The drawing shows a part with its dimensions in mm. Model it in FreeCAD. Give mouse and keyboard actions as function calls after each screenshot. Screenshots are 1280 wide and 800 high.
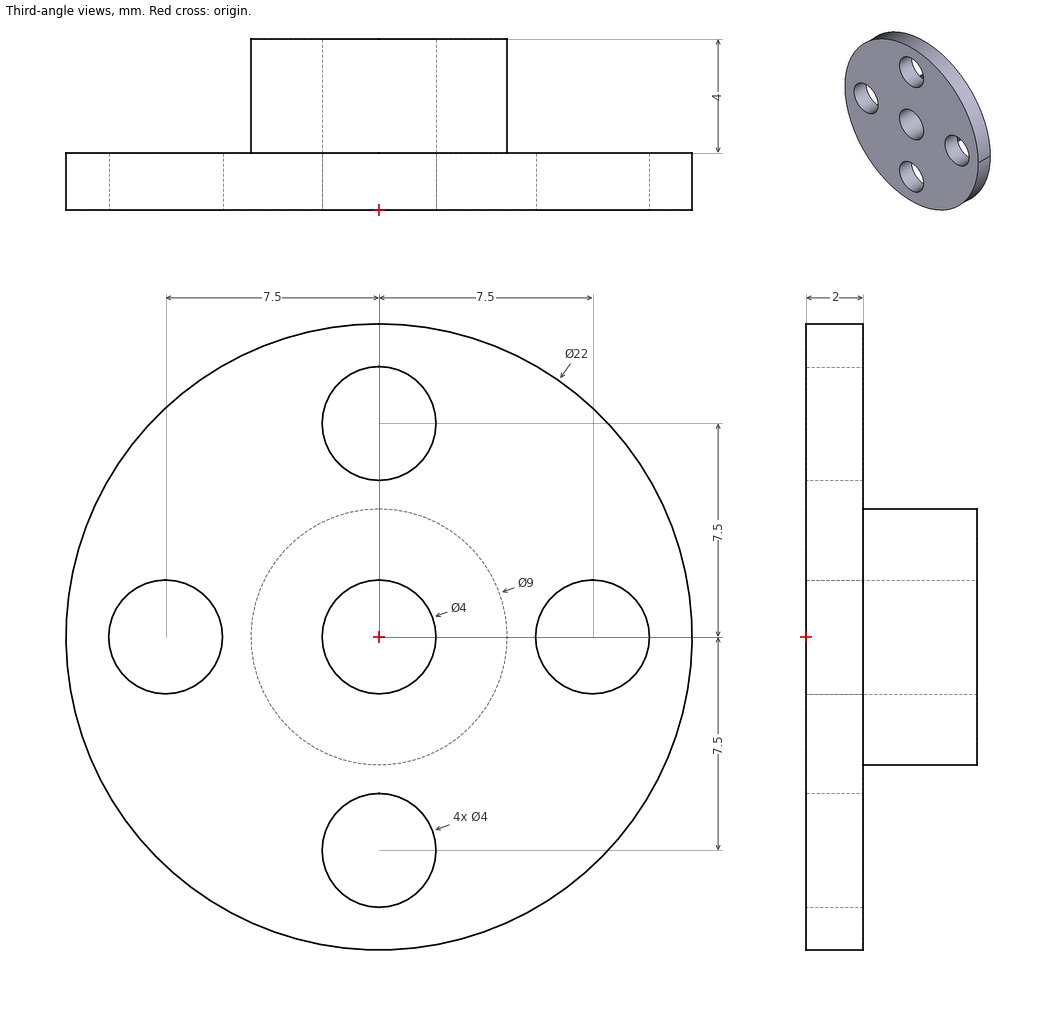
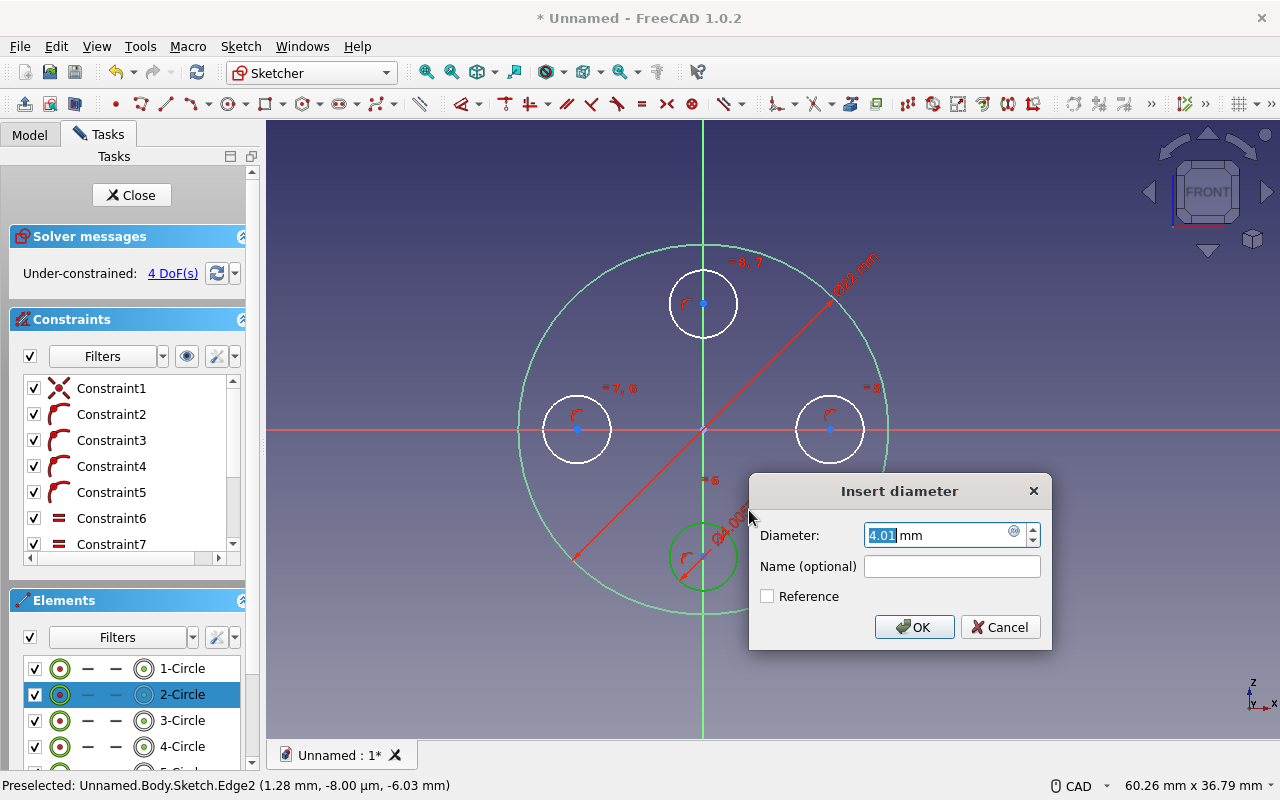
text(4)
key(Return)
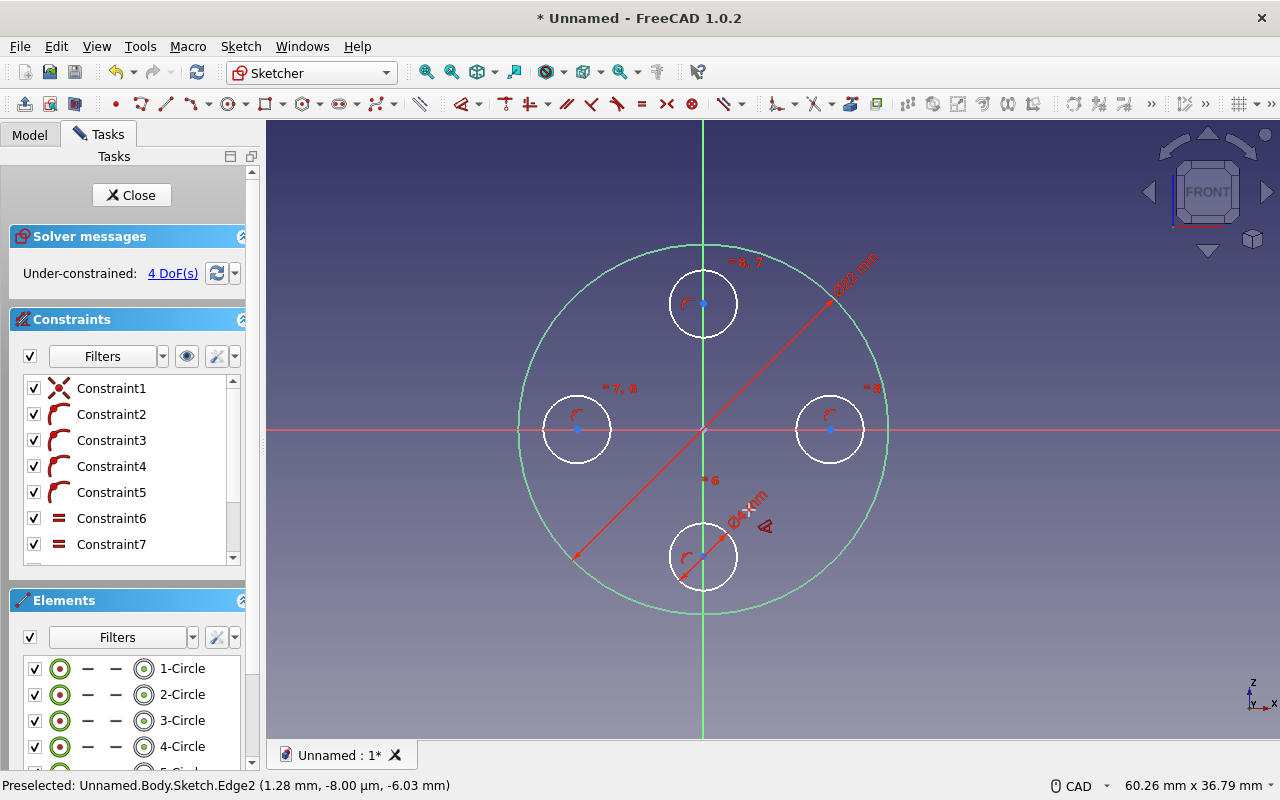
click(703, 557)
click(737, 464)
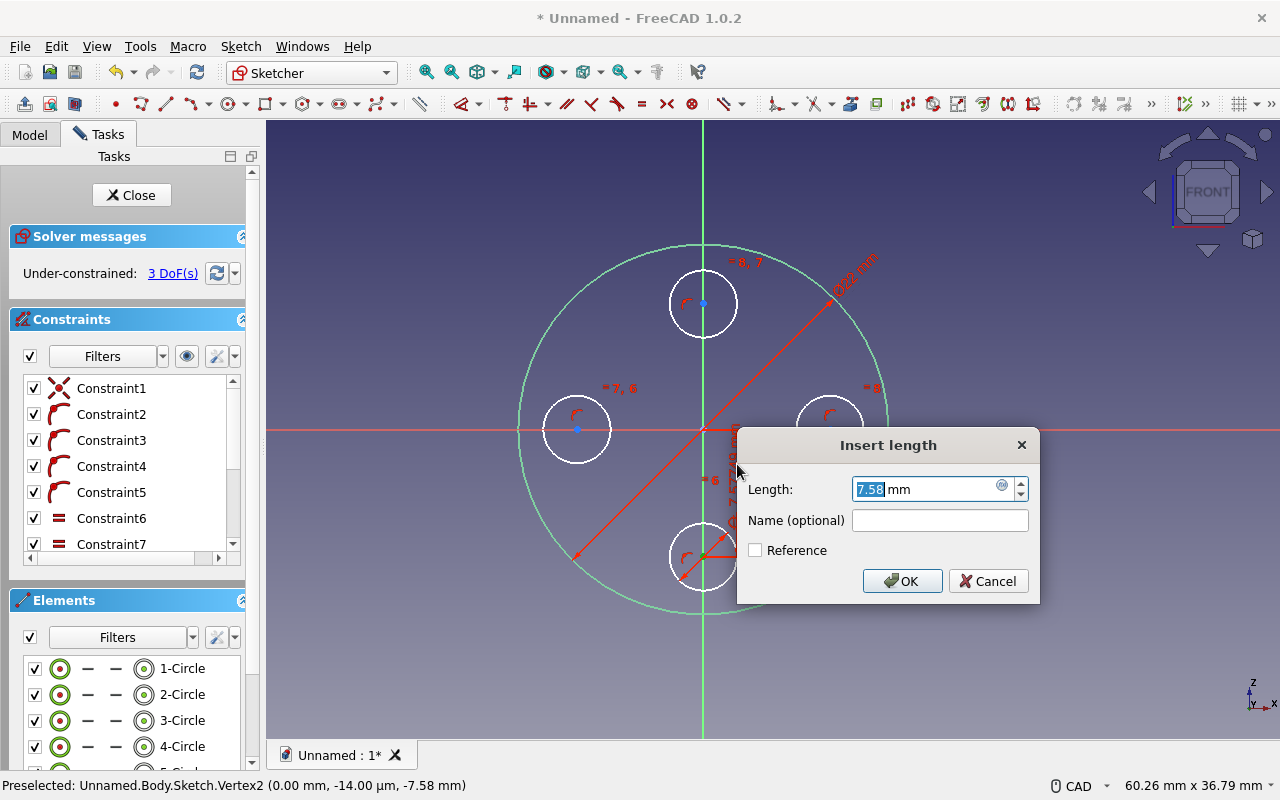
text(7.5)
key(Return)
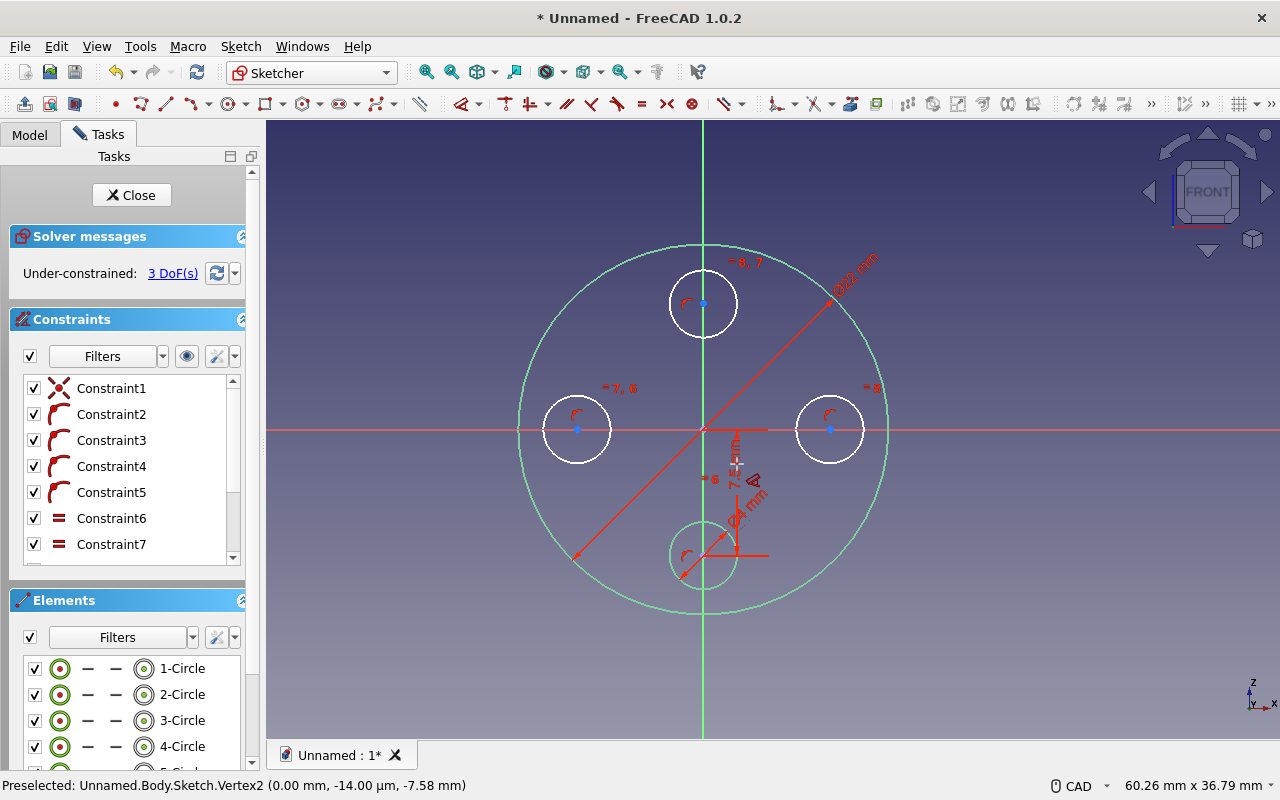
click(577, 430)
click(640, 464)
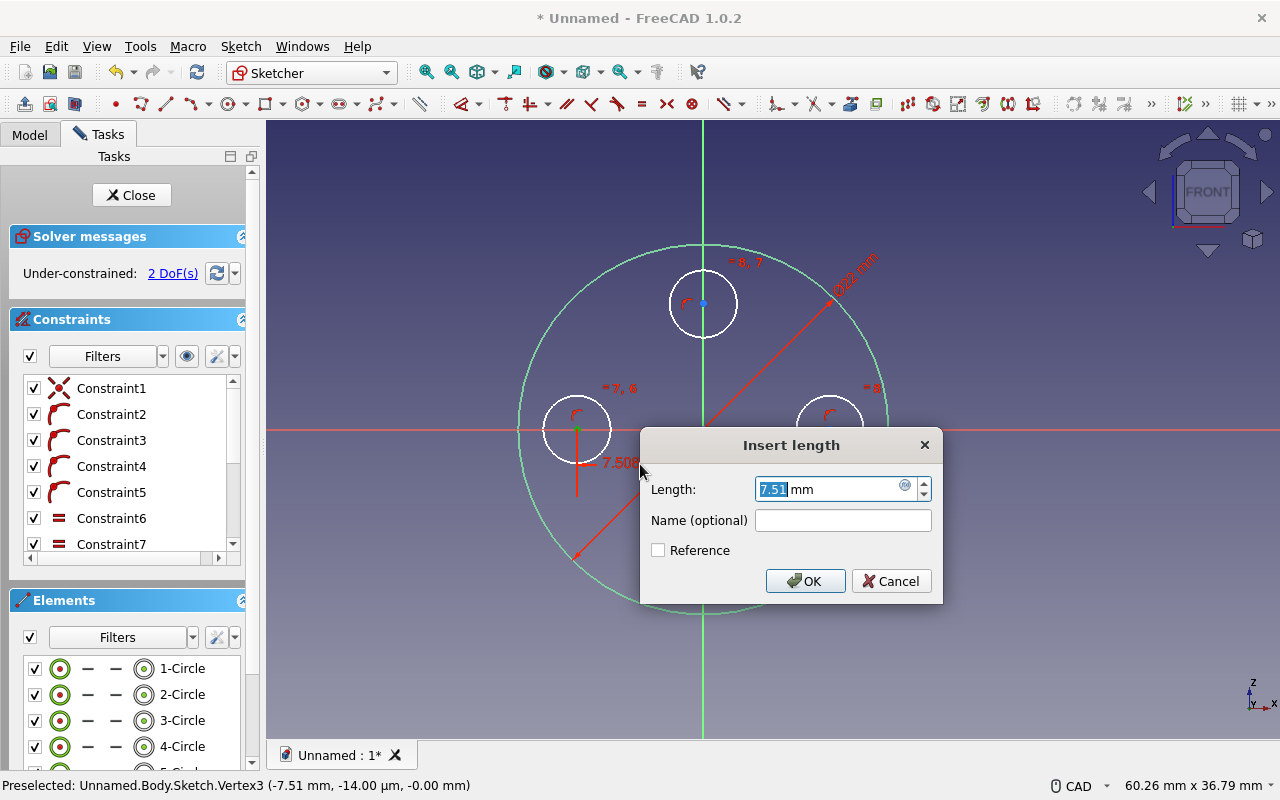
text(7.5)
key(Return)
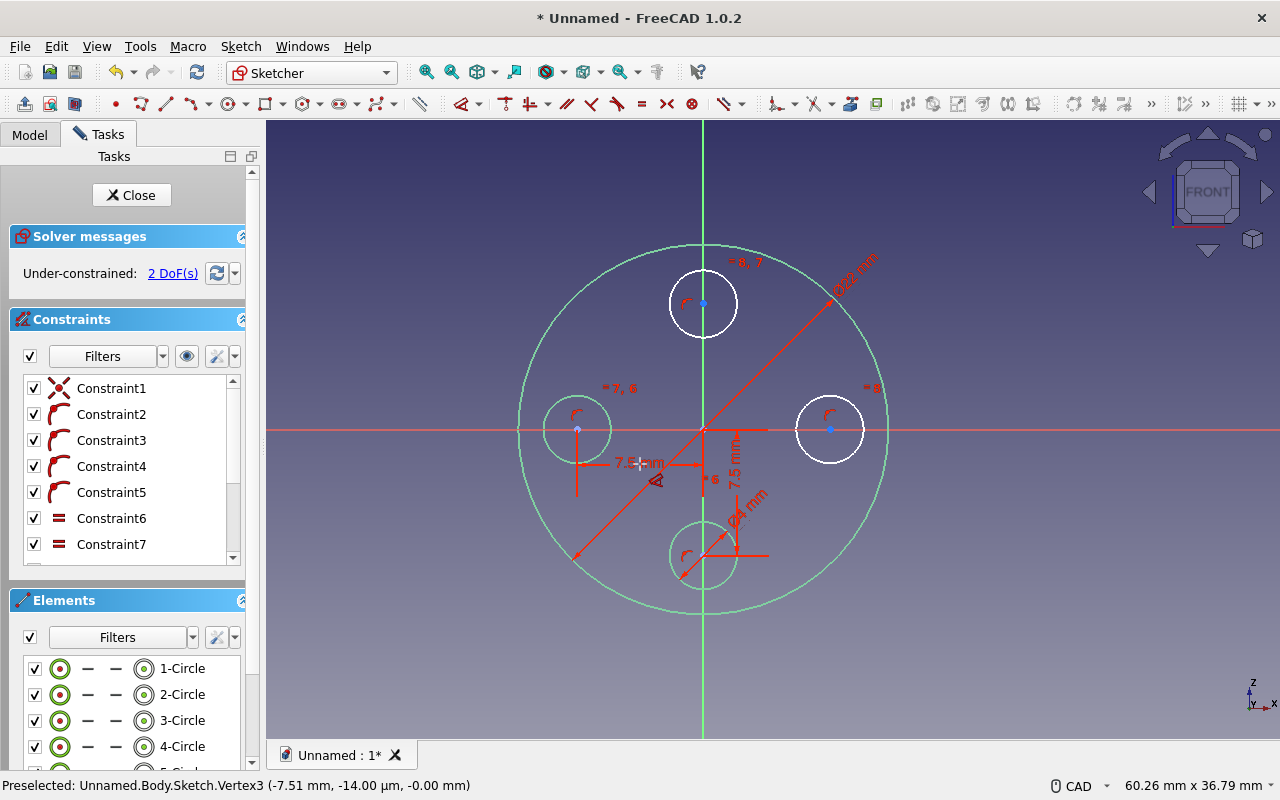
click(703, 304)
click(737, 367)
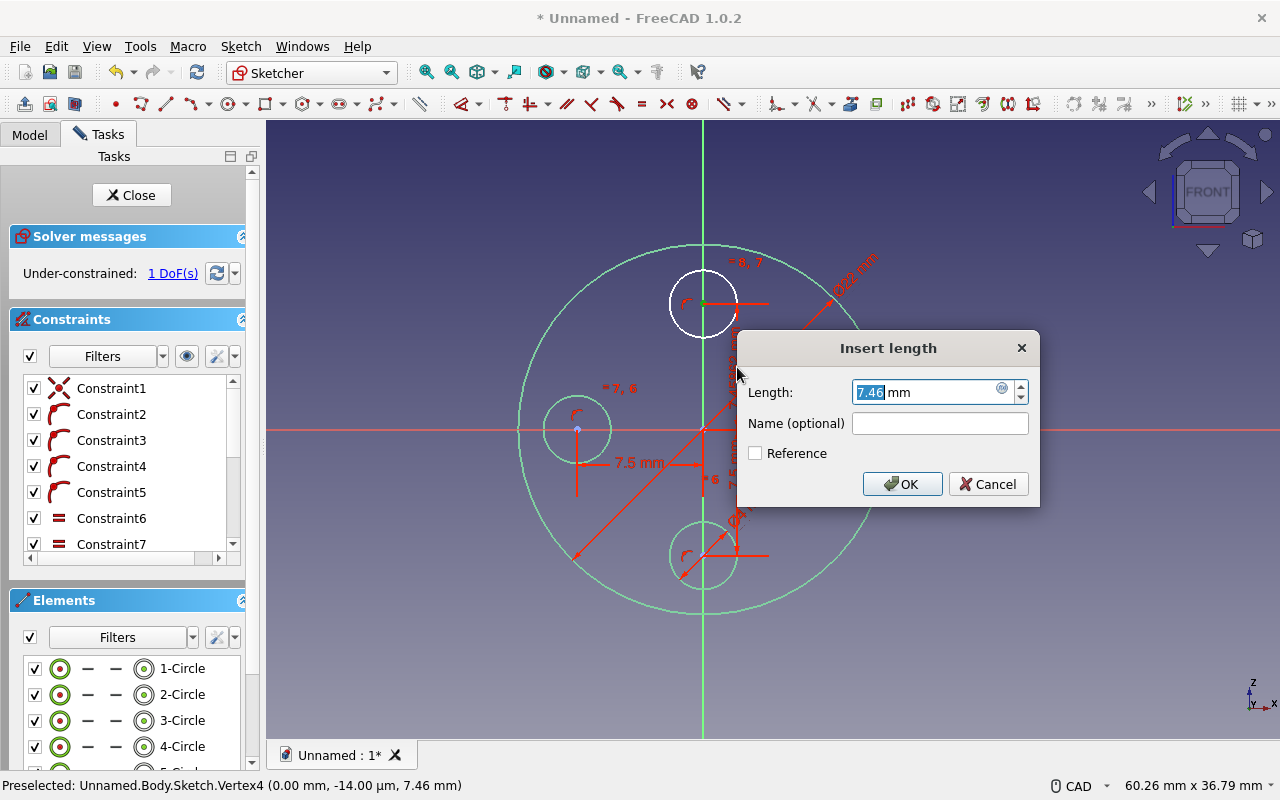
text(7.5)
key(Return)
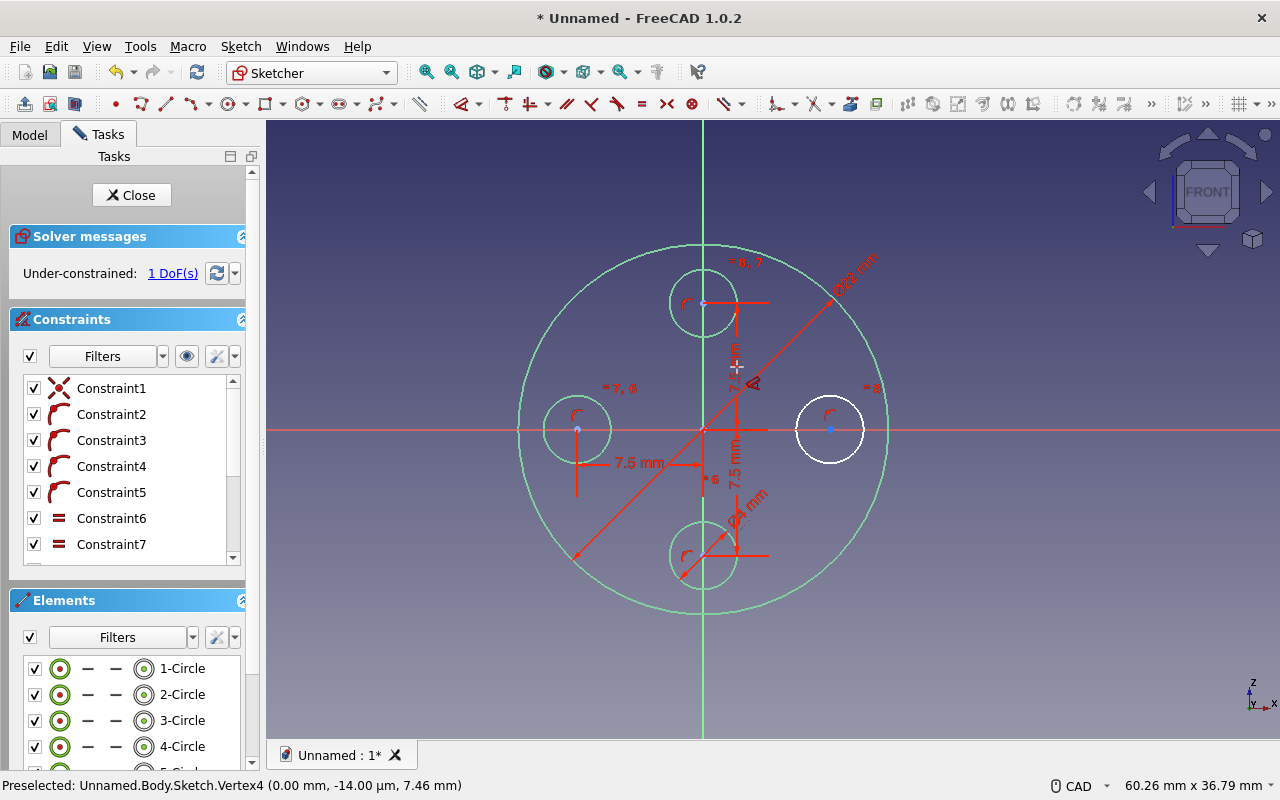
click(830, 430)
click(767, 396)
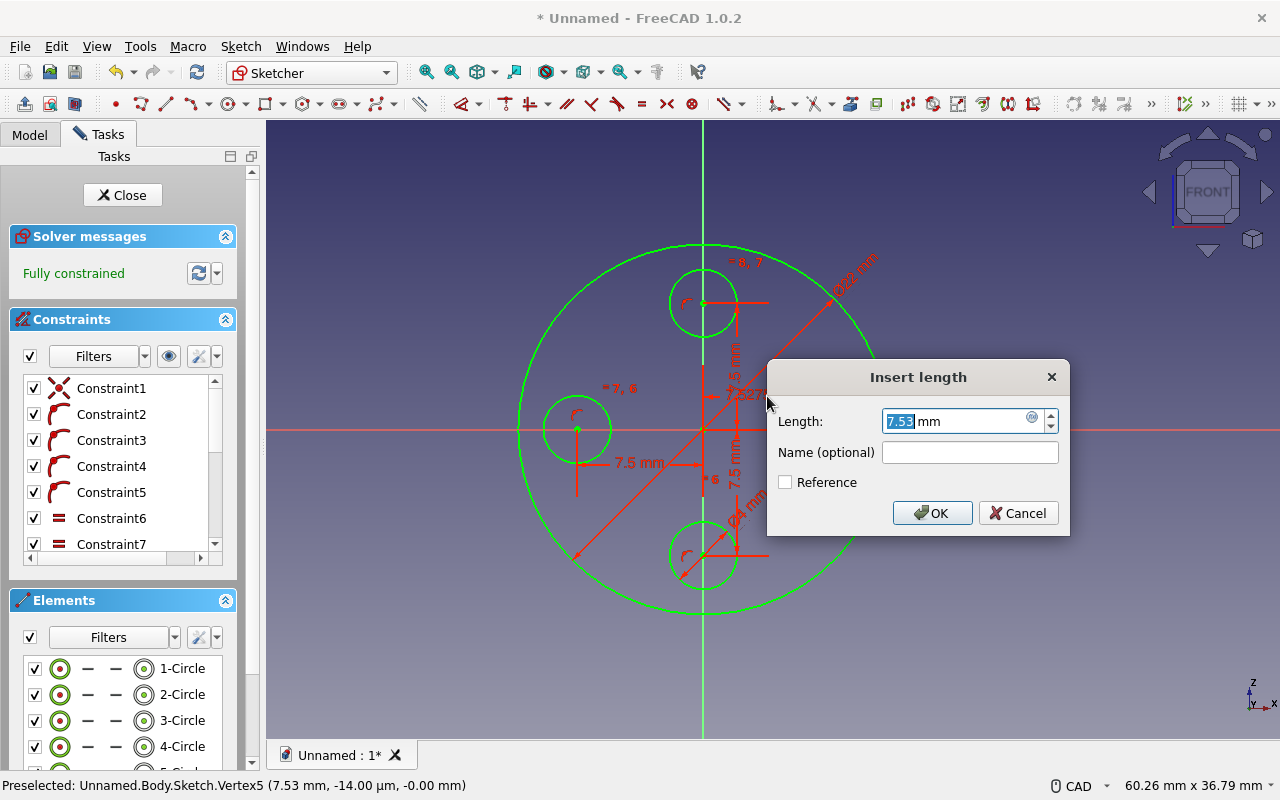
text(7.5)
key(Return)
key(Escape)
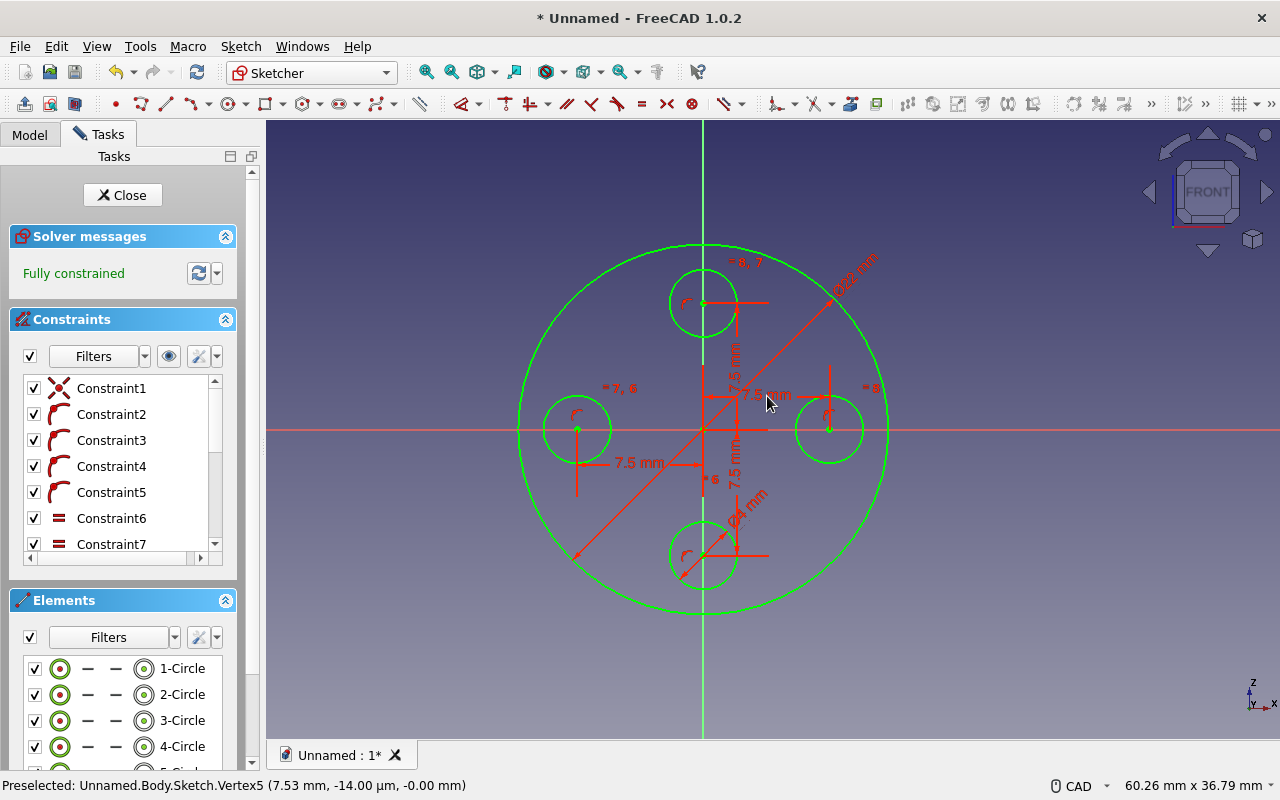
click(123, 195)